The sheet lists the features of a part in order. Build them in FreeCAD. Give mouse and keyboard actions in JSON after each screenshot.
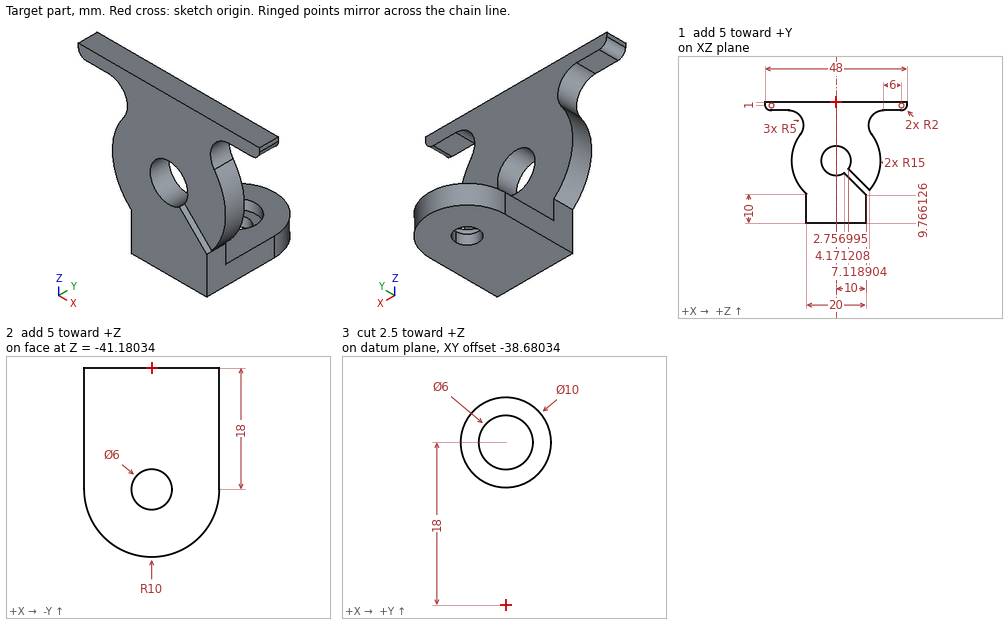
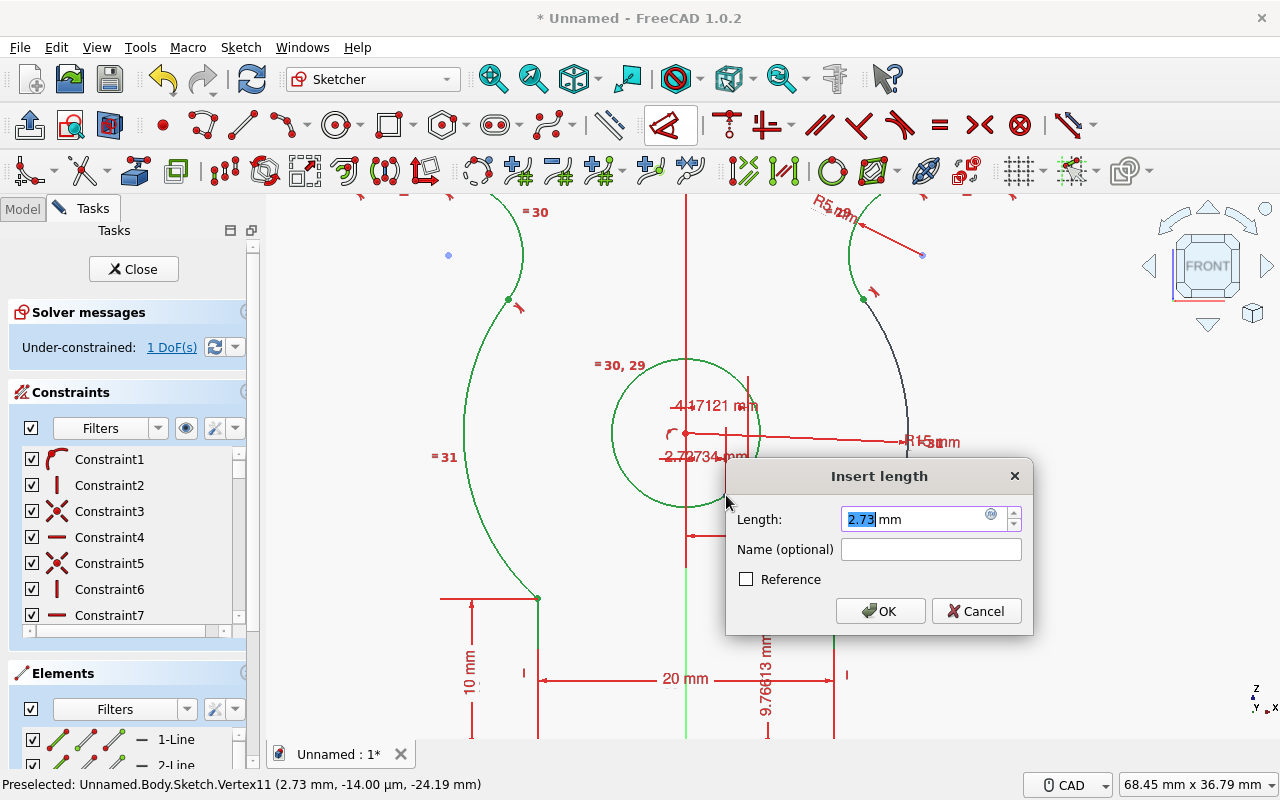
{"action": "type", "text": "2.756995"}
{"action": "key", "text": "Return"}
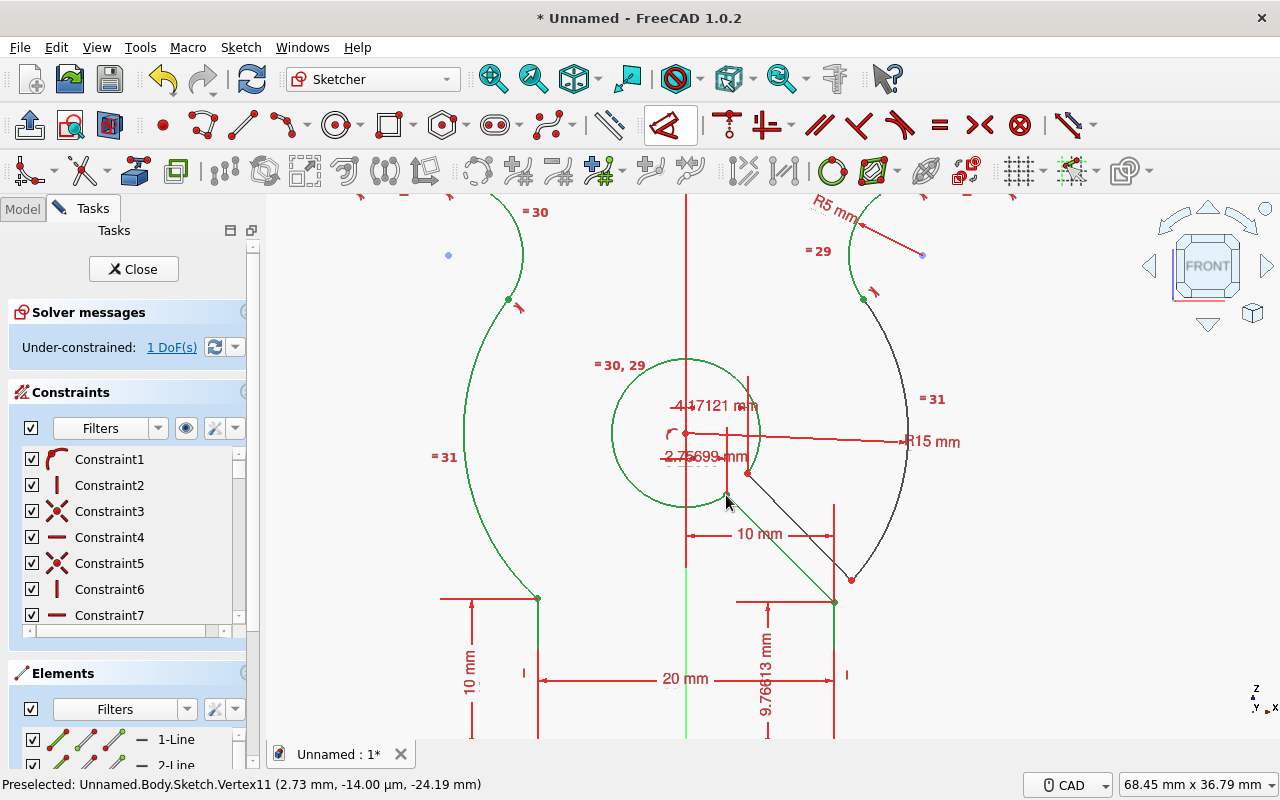
{"action": "left_click", "coordinate": [821, 549]}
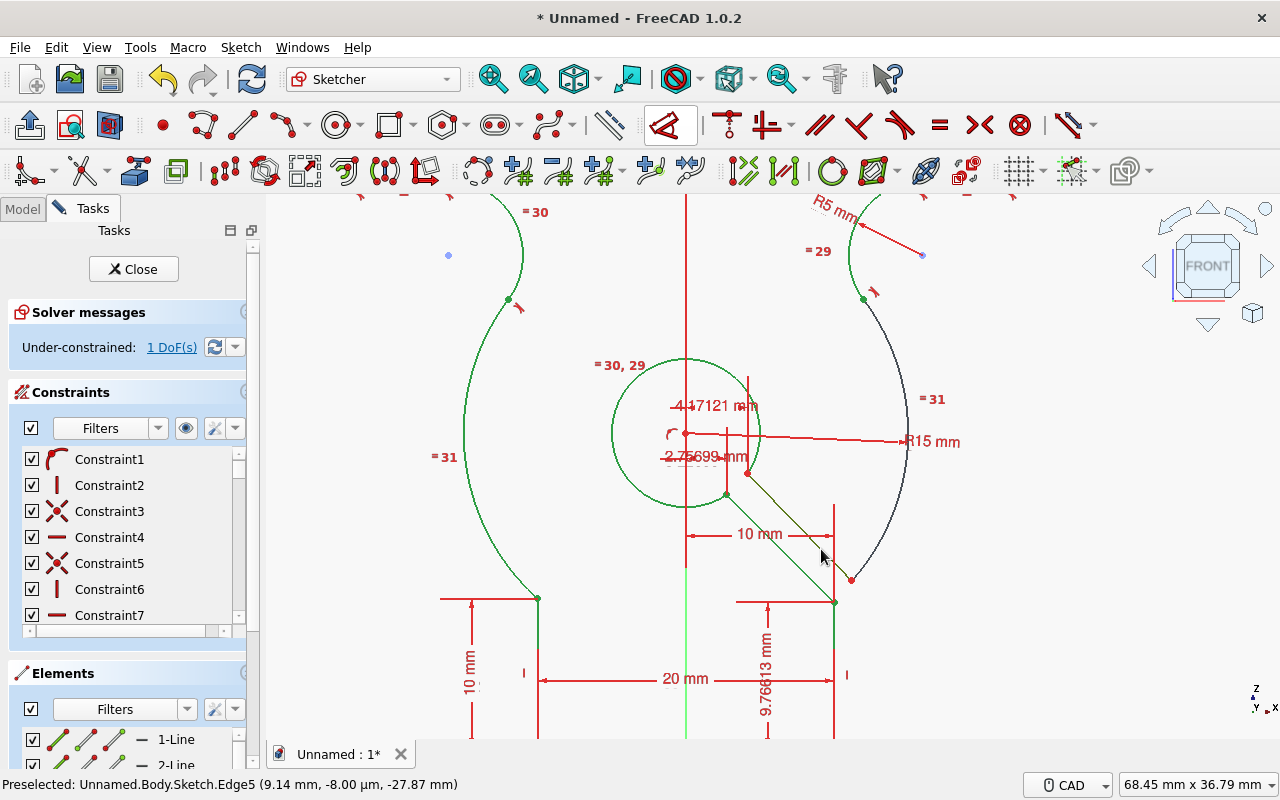
{"action": "key", "text": "l"}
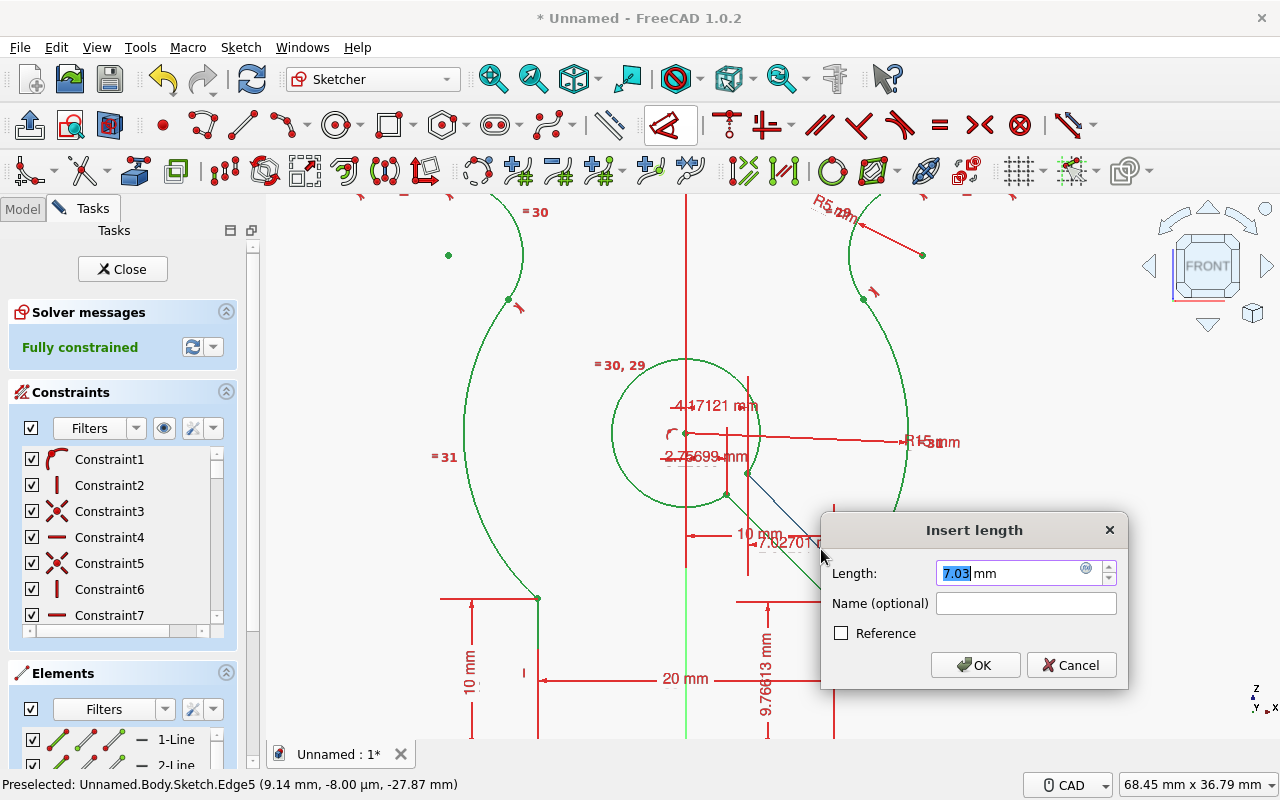
{"action": "type", "text": "7.118904"}
{"action": "key", "text": "Return"}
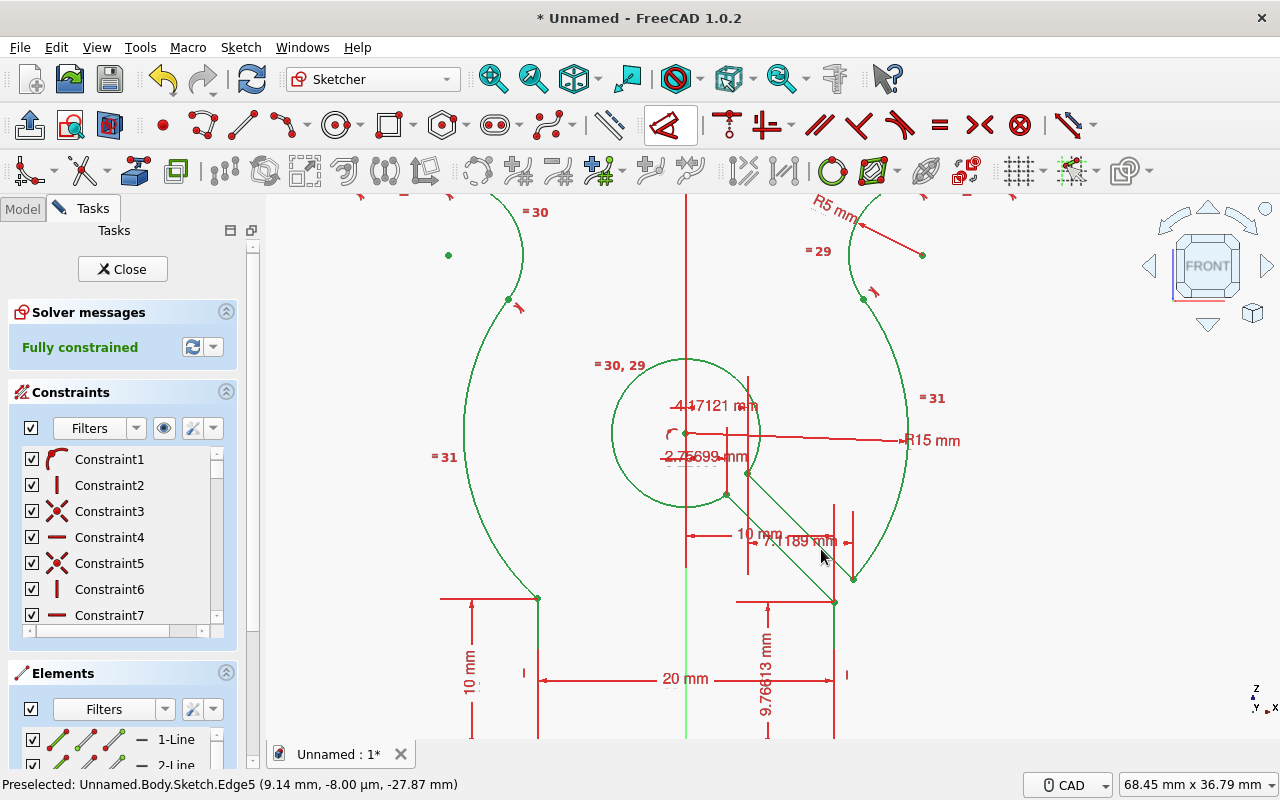
{"action": "left_click", "coordinate": [123, 269]}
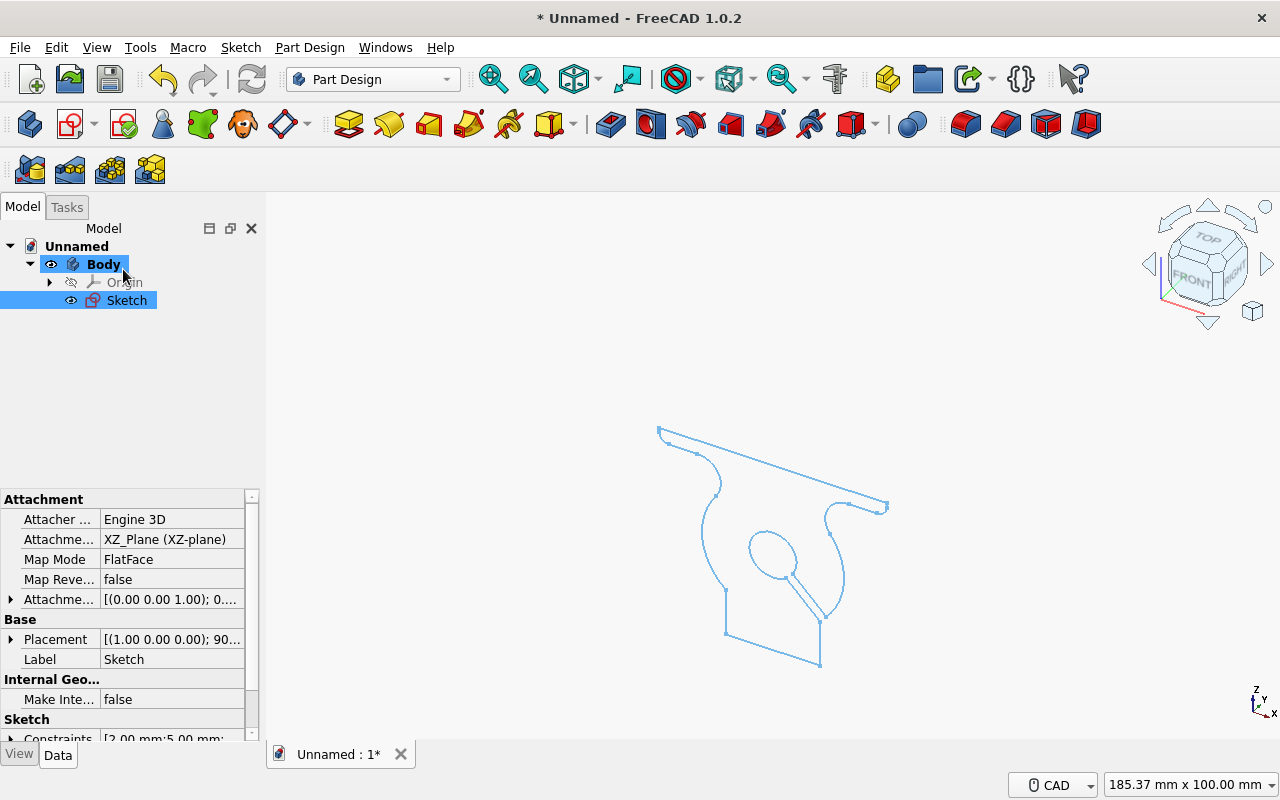
{"action": "left_click", "coordinate": [350, 124]}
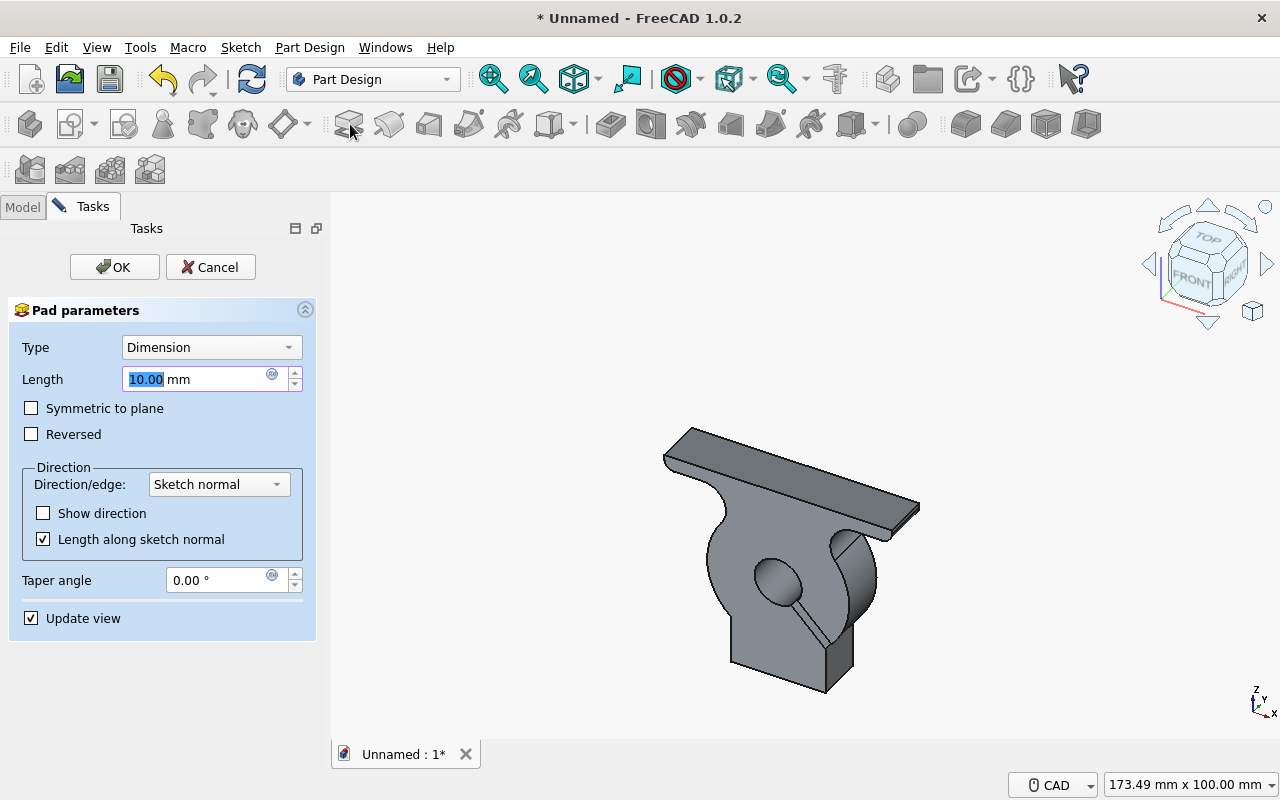
{"action": "type", "text": "5"}
{"action": "key", "text": "Tab"}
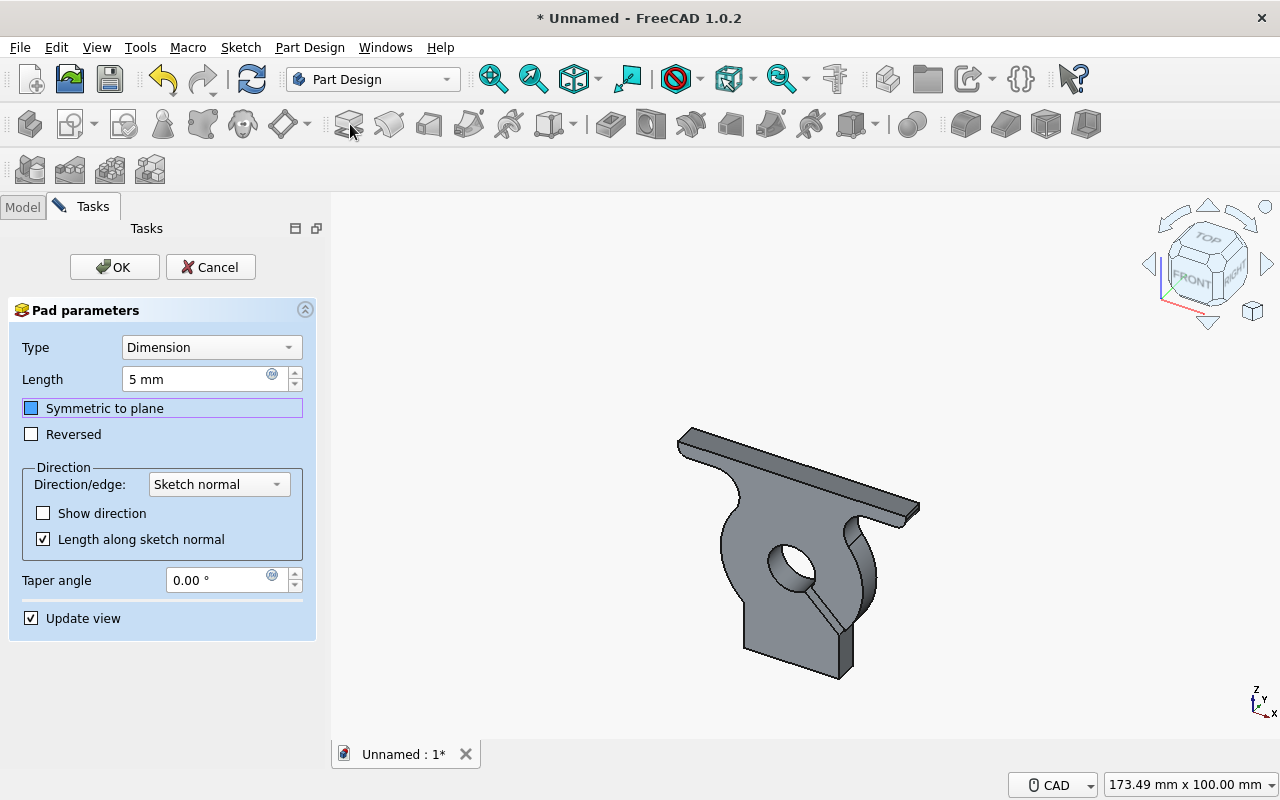
{"action": "left_click", "coordinate": [30, 434]}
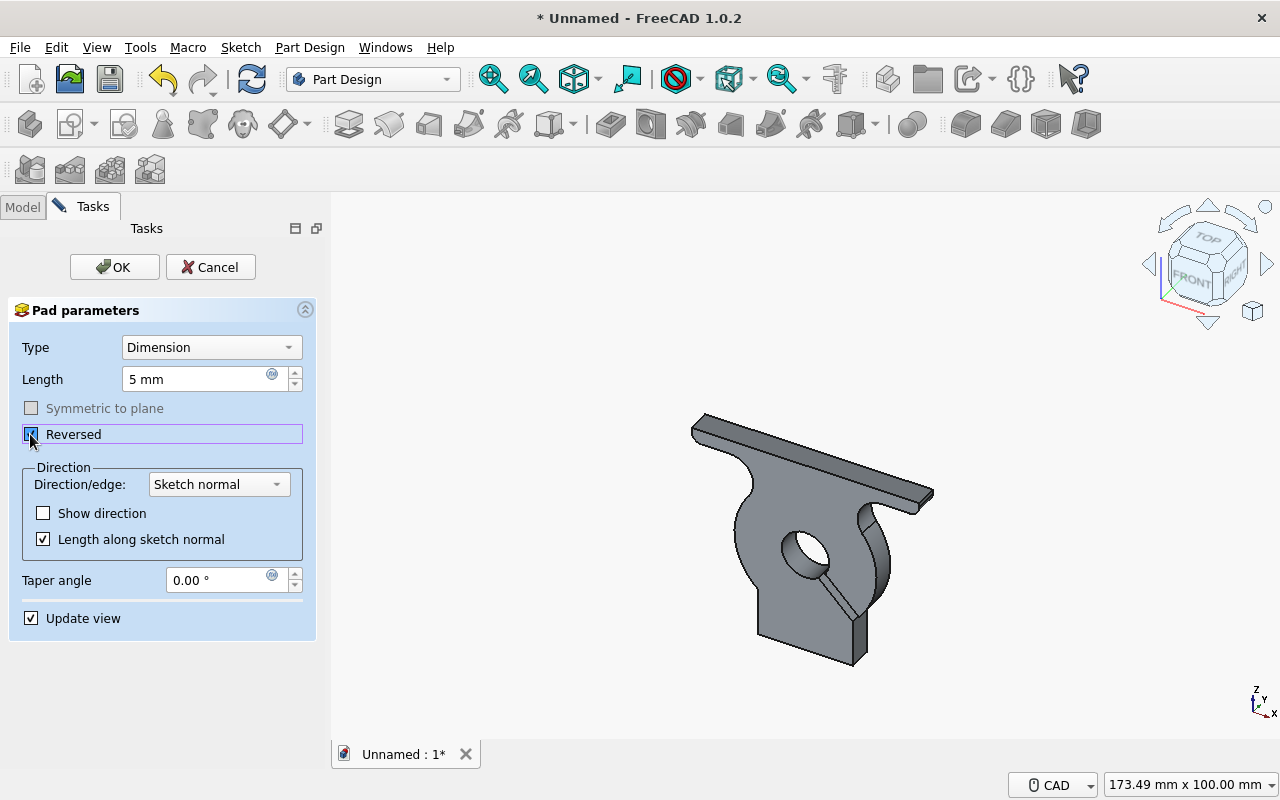
{"action": "left_click", "coordinate": [115, 267]}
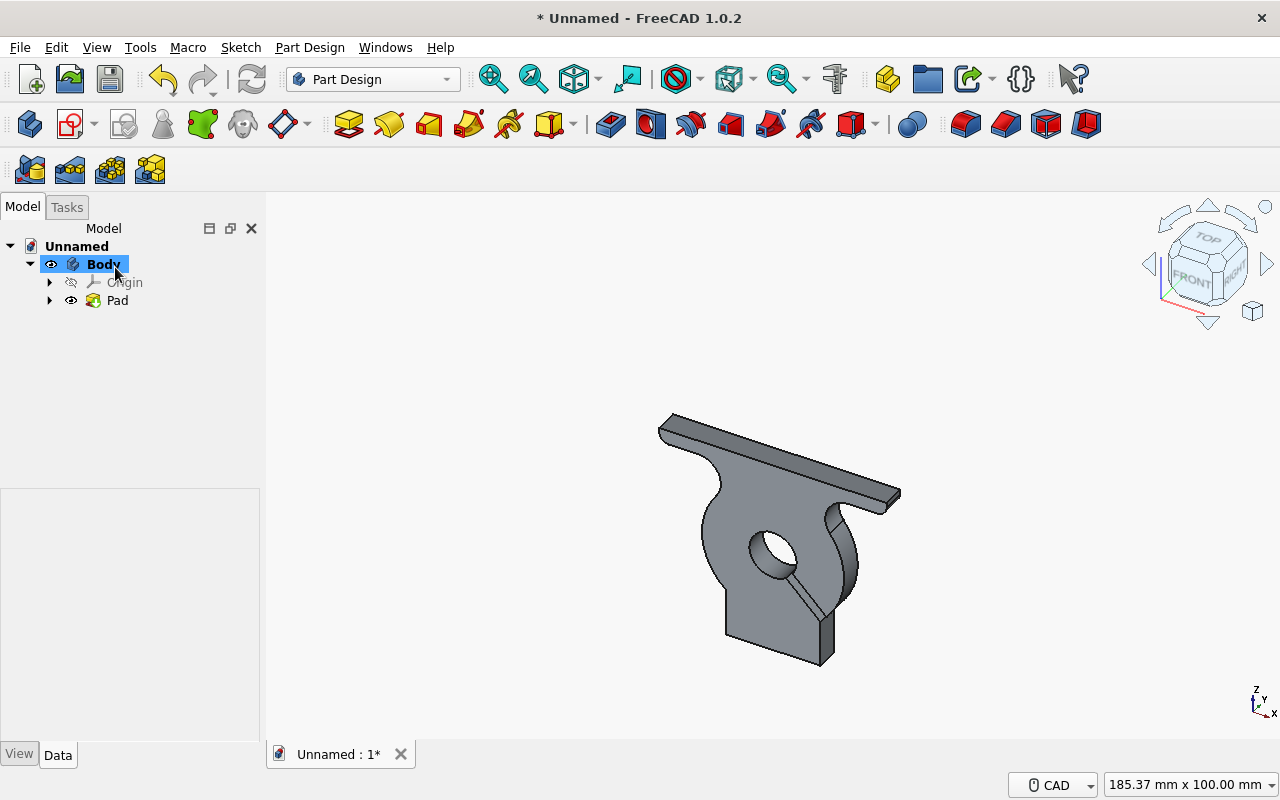
{"action": "key", "text": "5"}